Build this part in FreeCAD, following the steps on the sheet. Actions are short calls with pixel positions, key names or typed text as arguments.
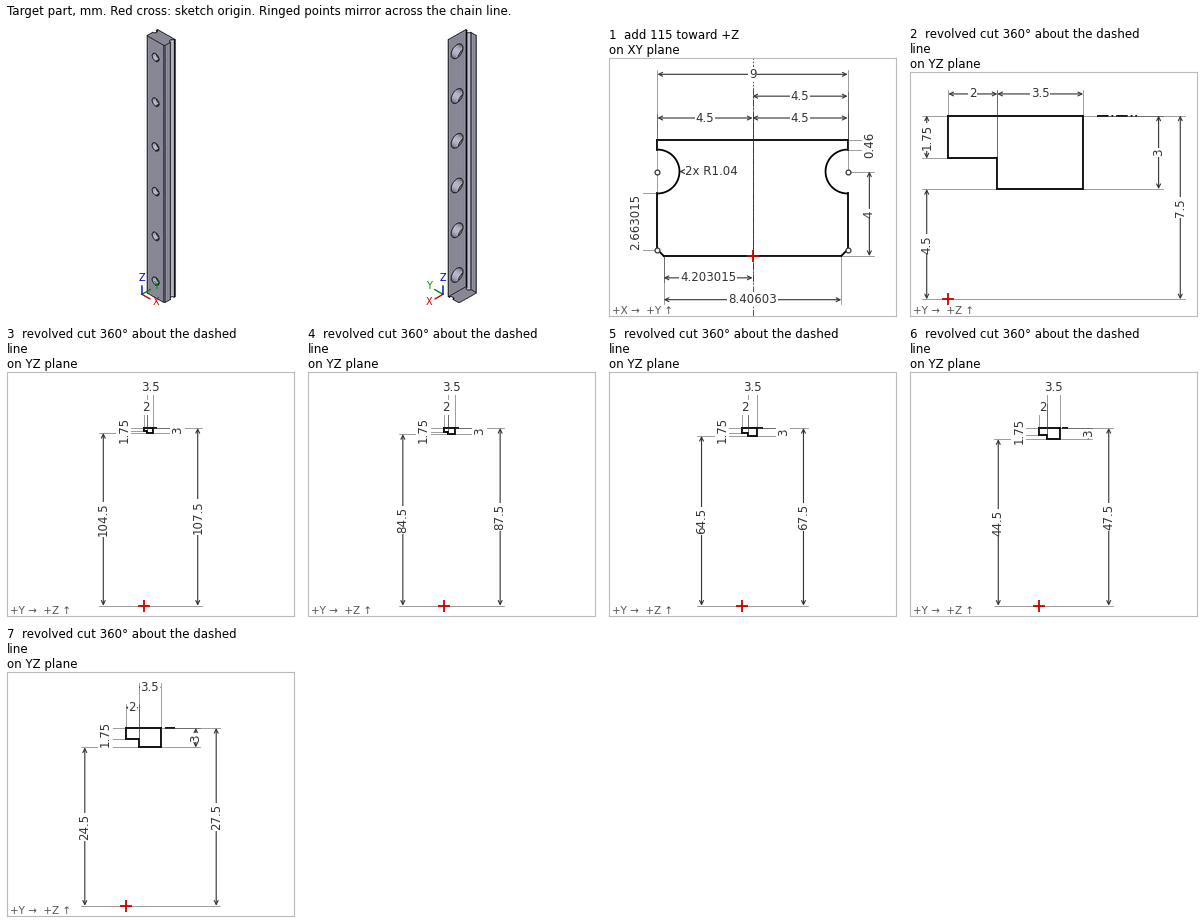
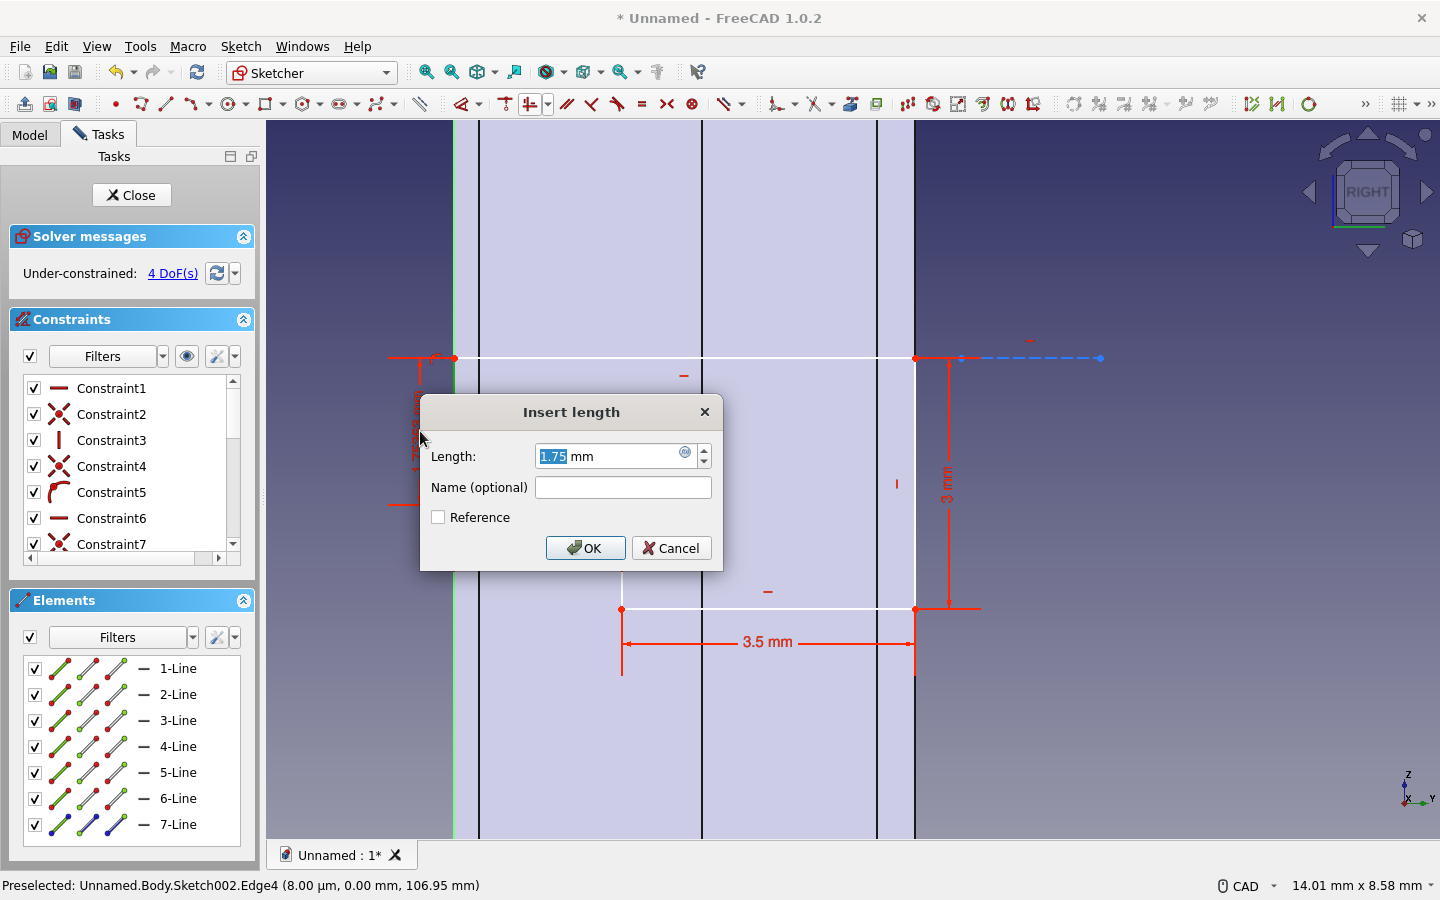
text(1.75)
key(Return)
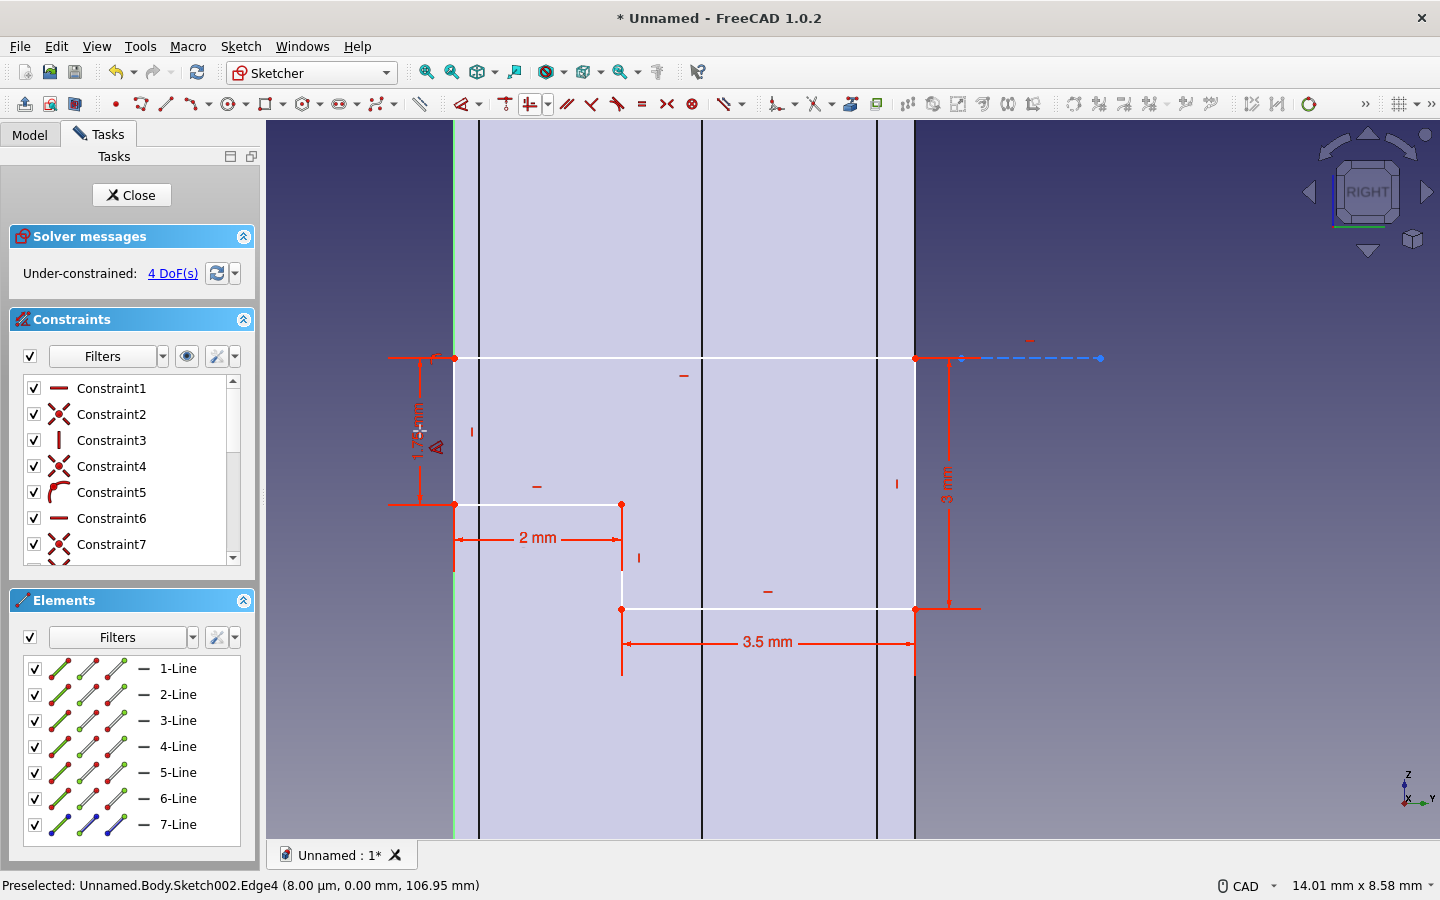
click(622, 609)
click(420, 710)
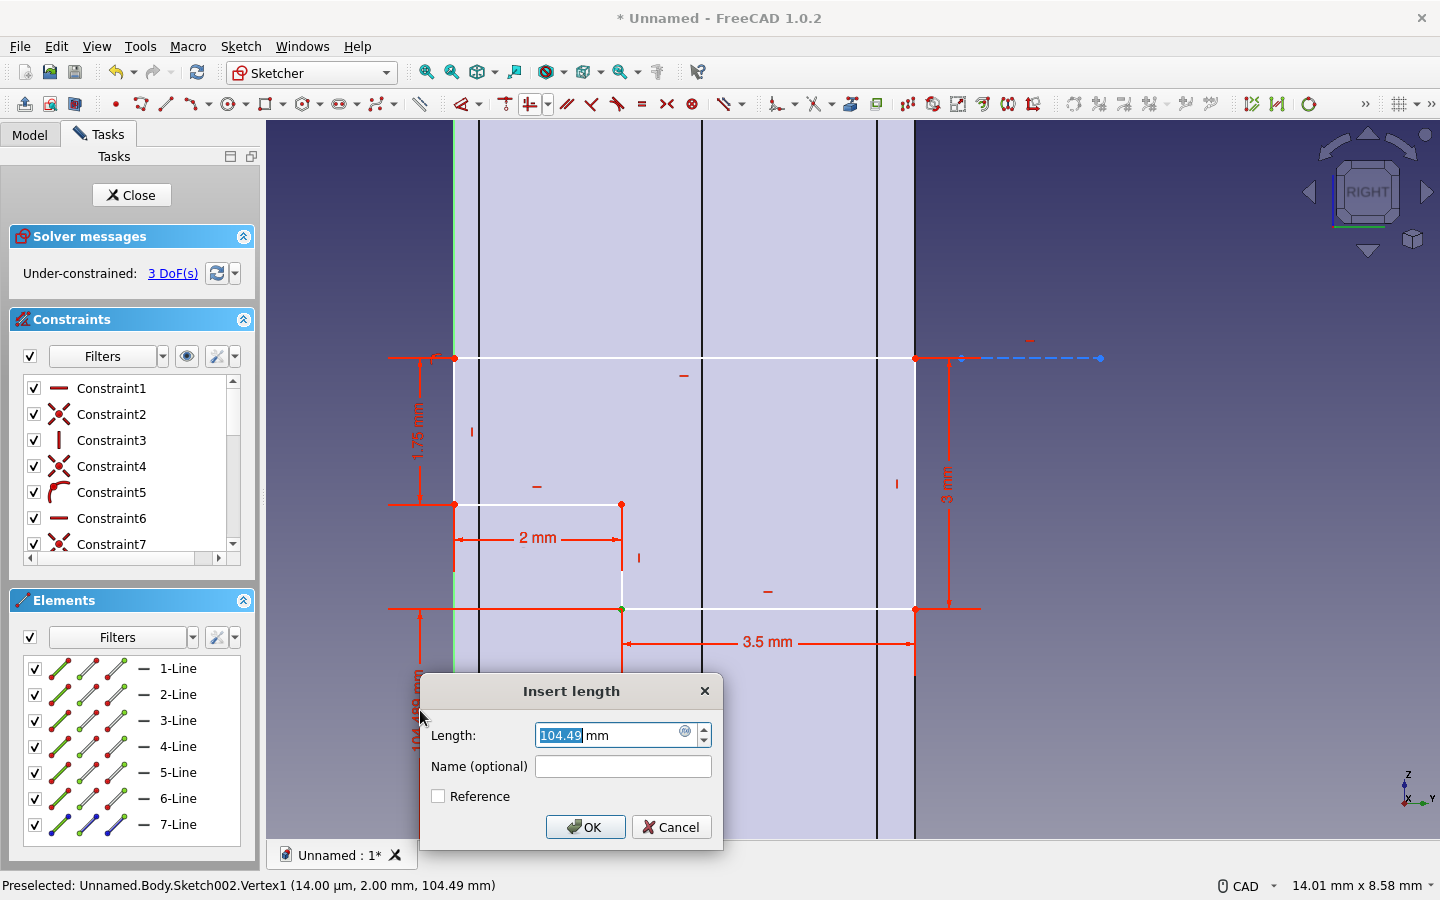
text(104.5)
key(Return)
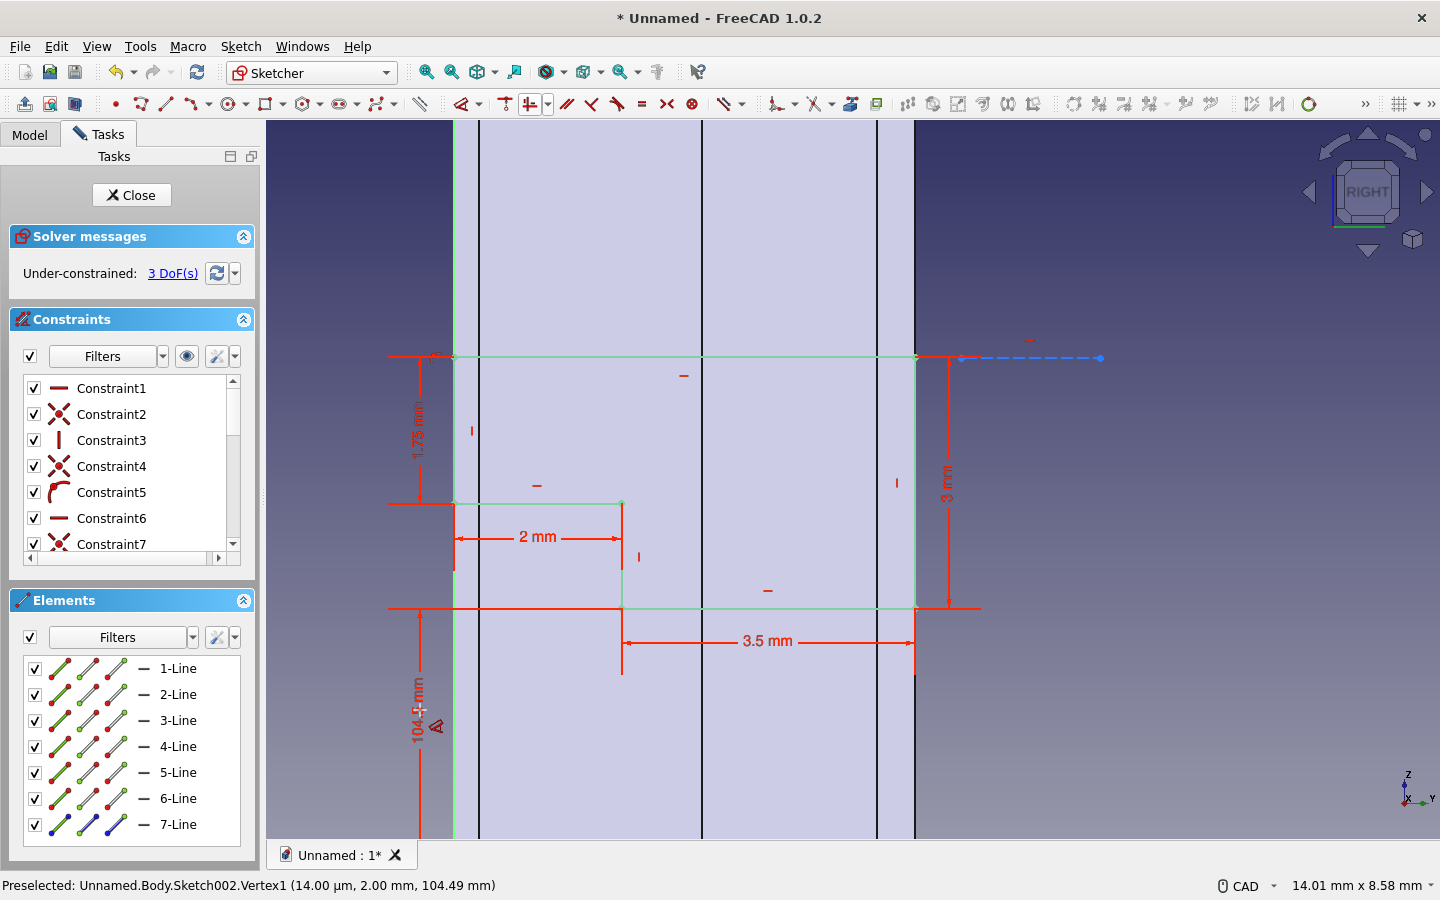
click(961, 358)
click(420, 585)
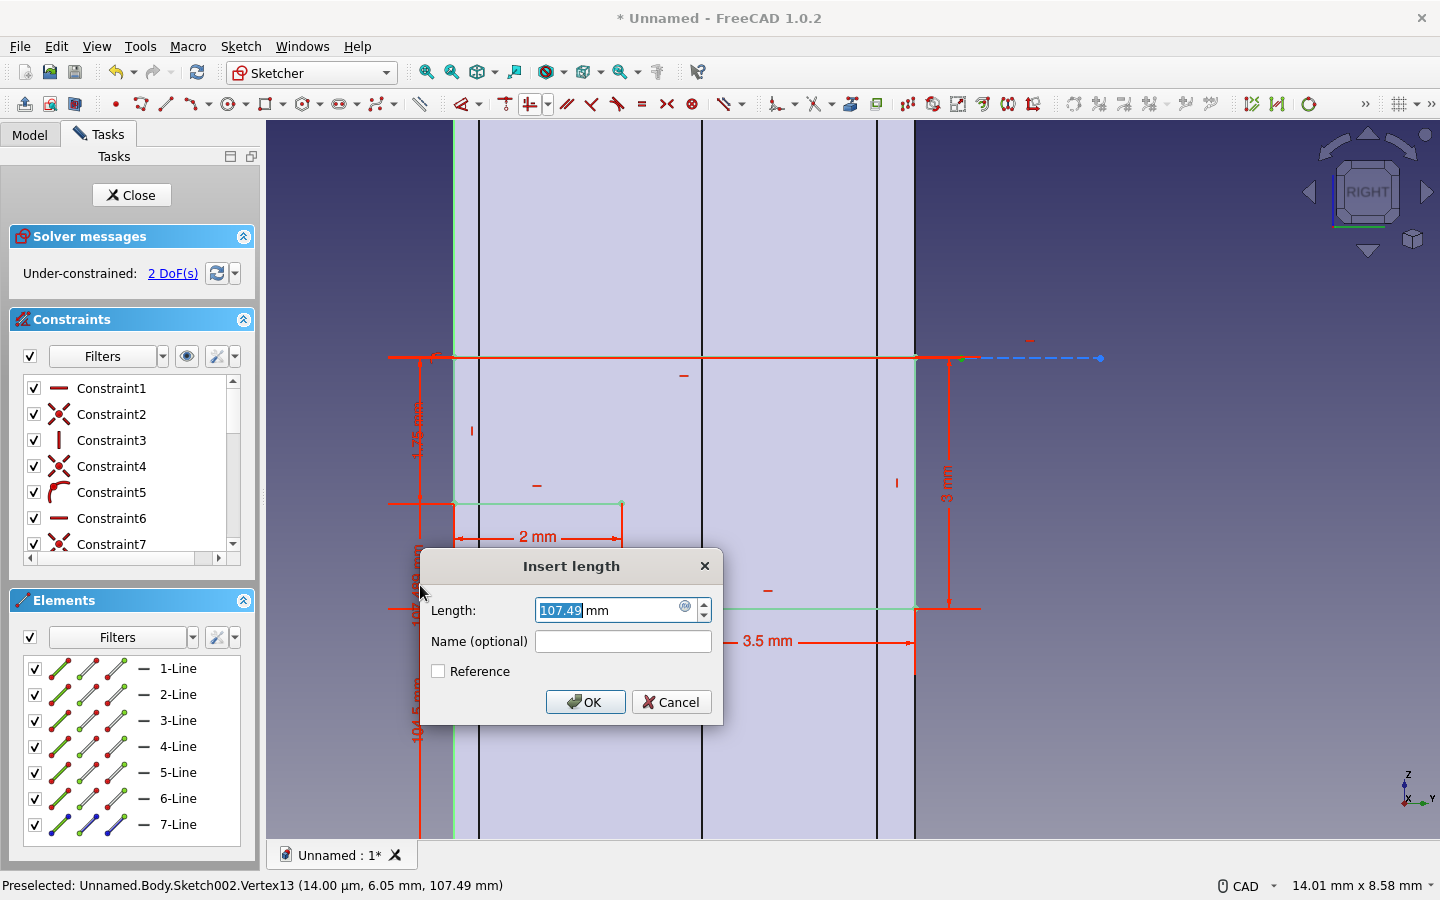
text(107.5)
key(Return)
key(Escape)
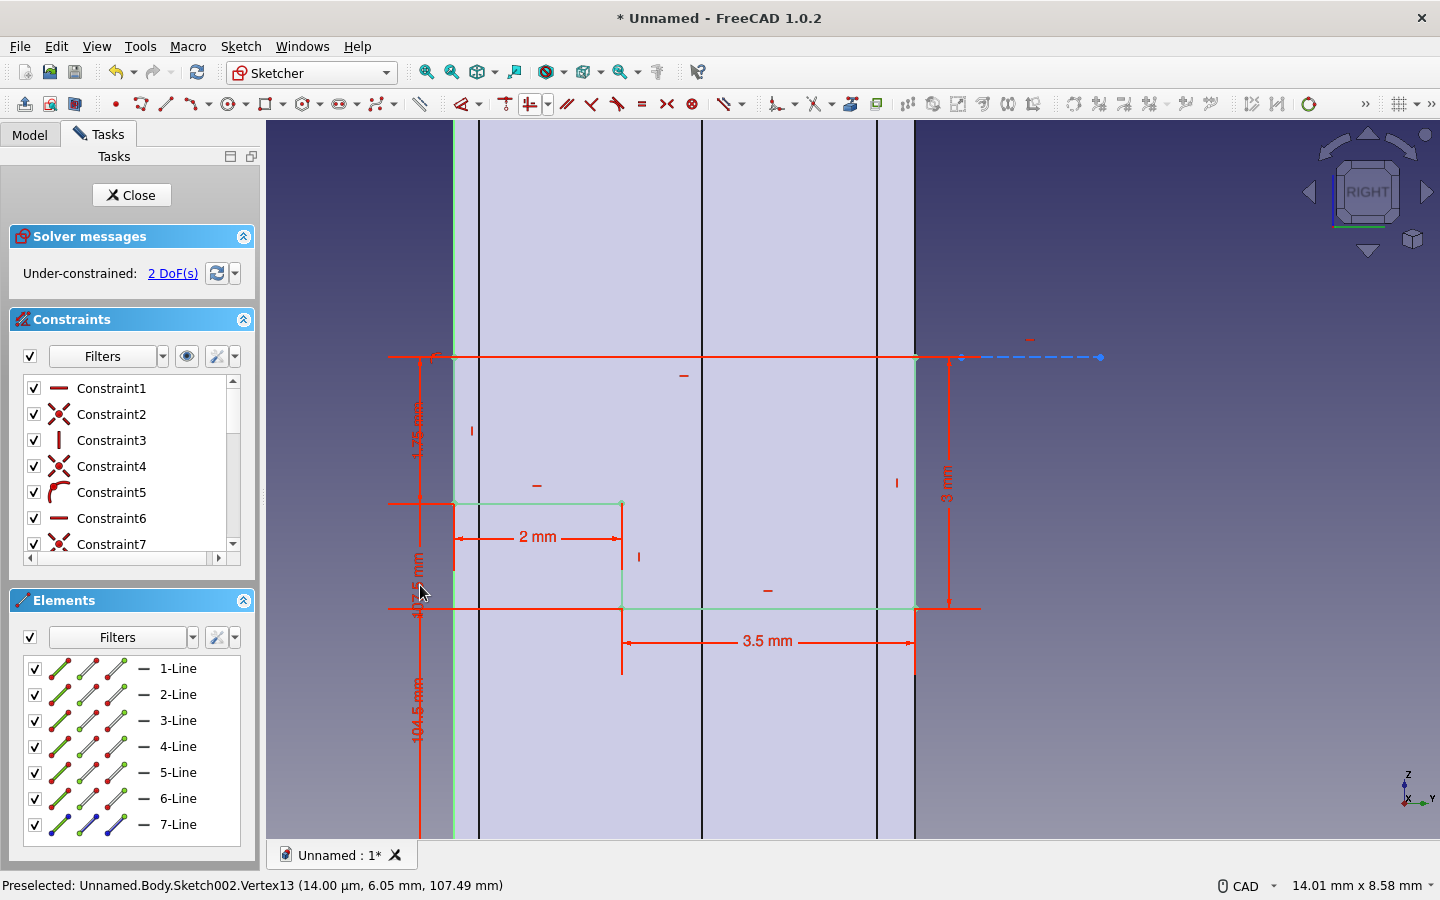
click(132, 195)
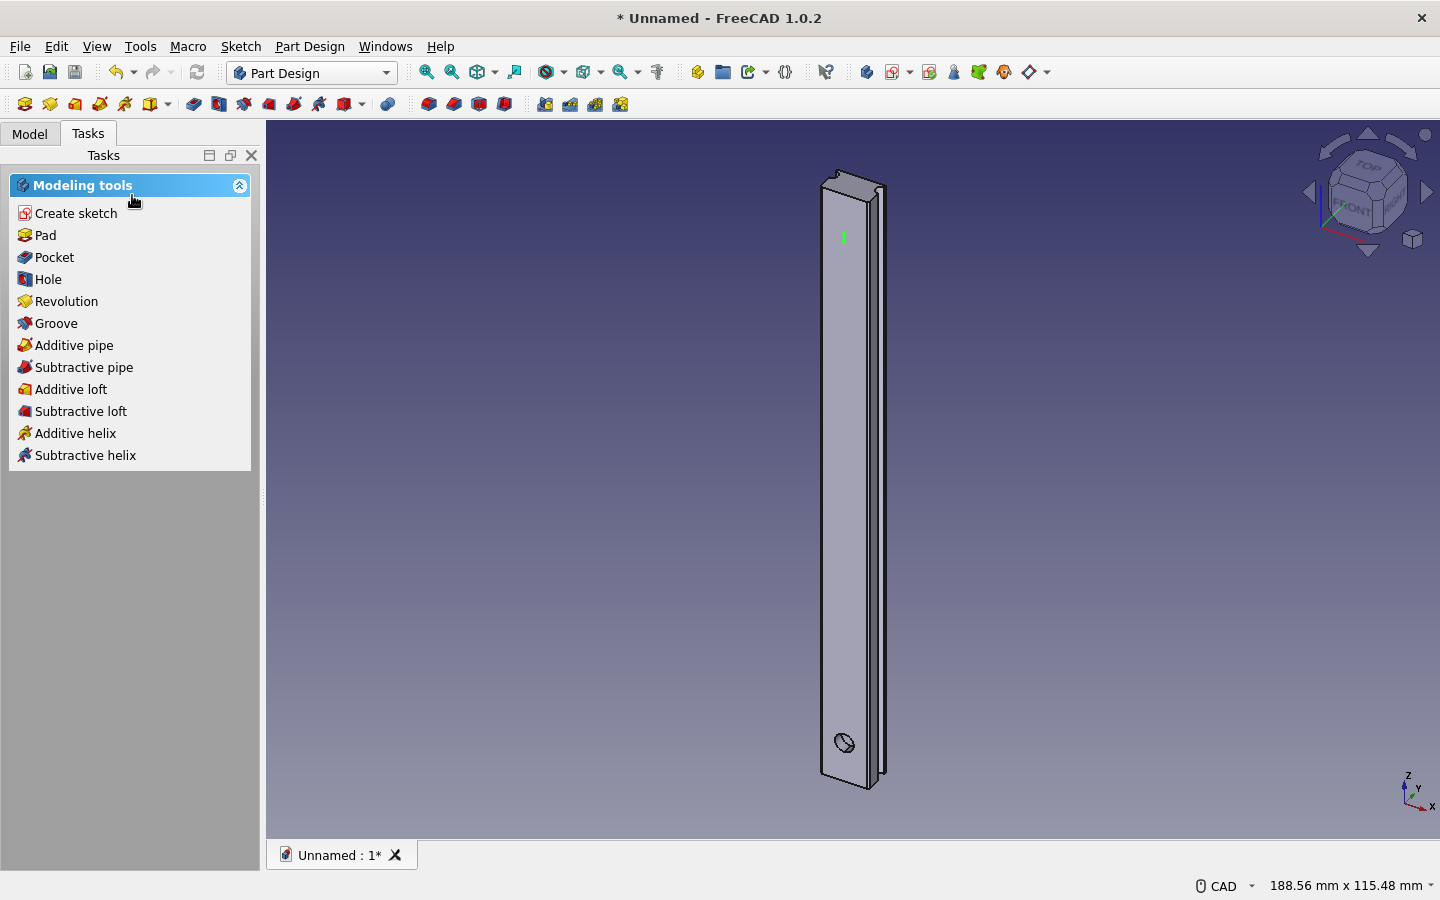
click(244, 104)